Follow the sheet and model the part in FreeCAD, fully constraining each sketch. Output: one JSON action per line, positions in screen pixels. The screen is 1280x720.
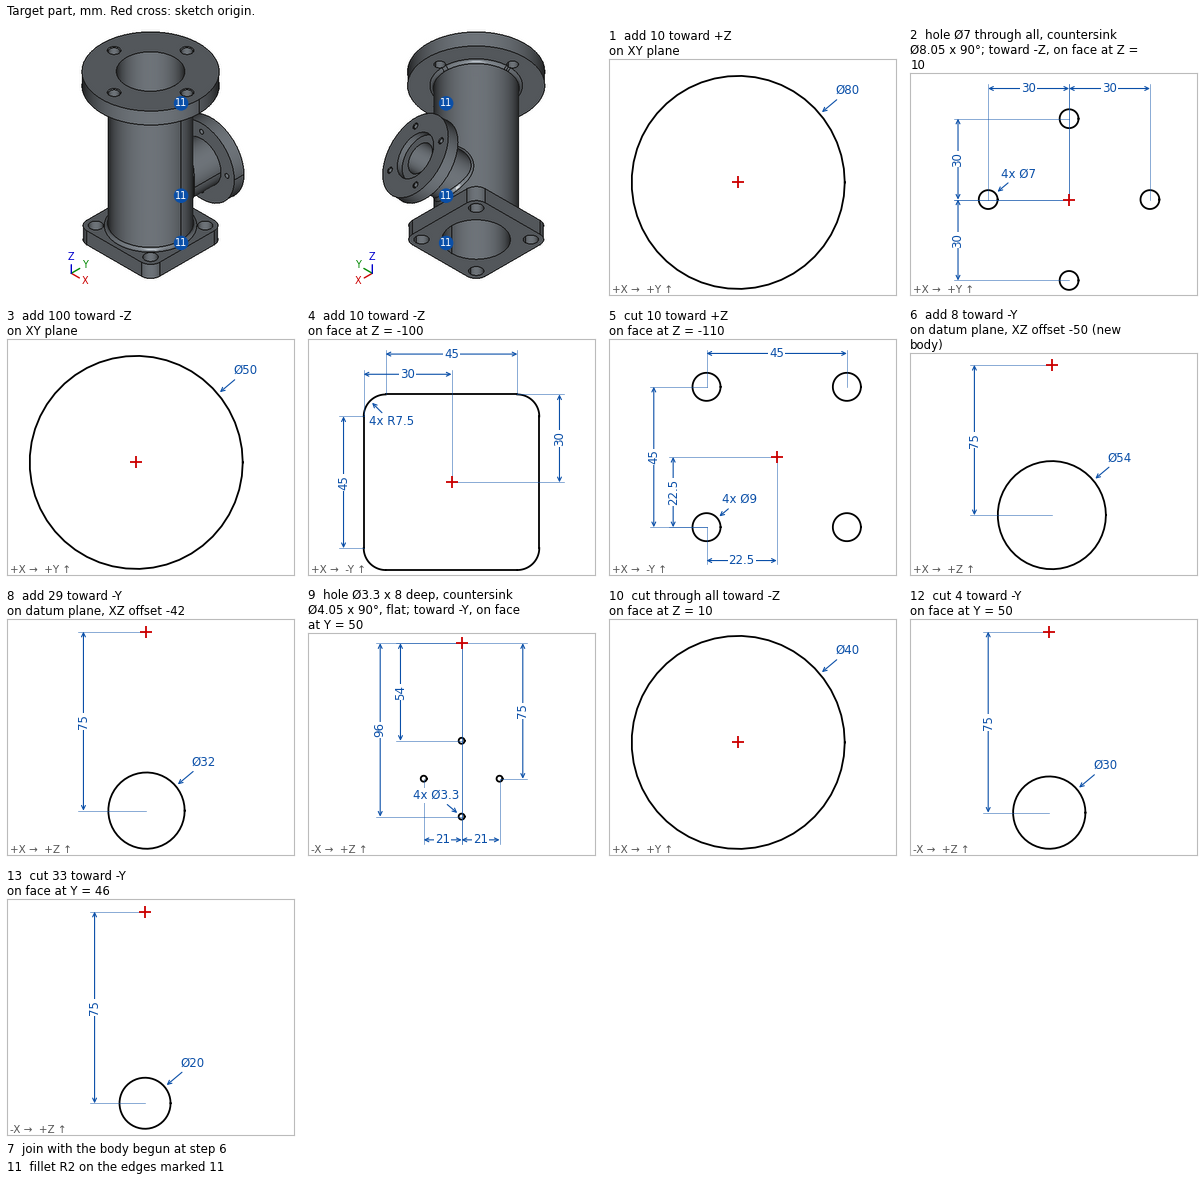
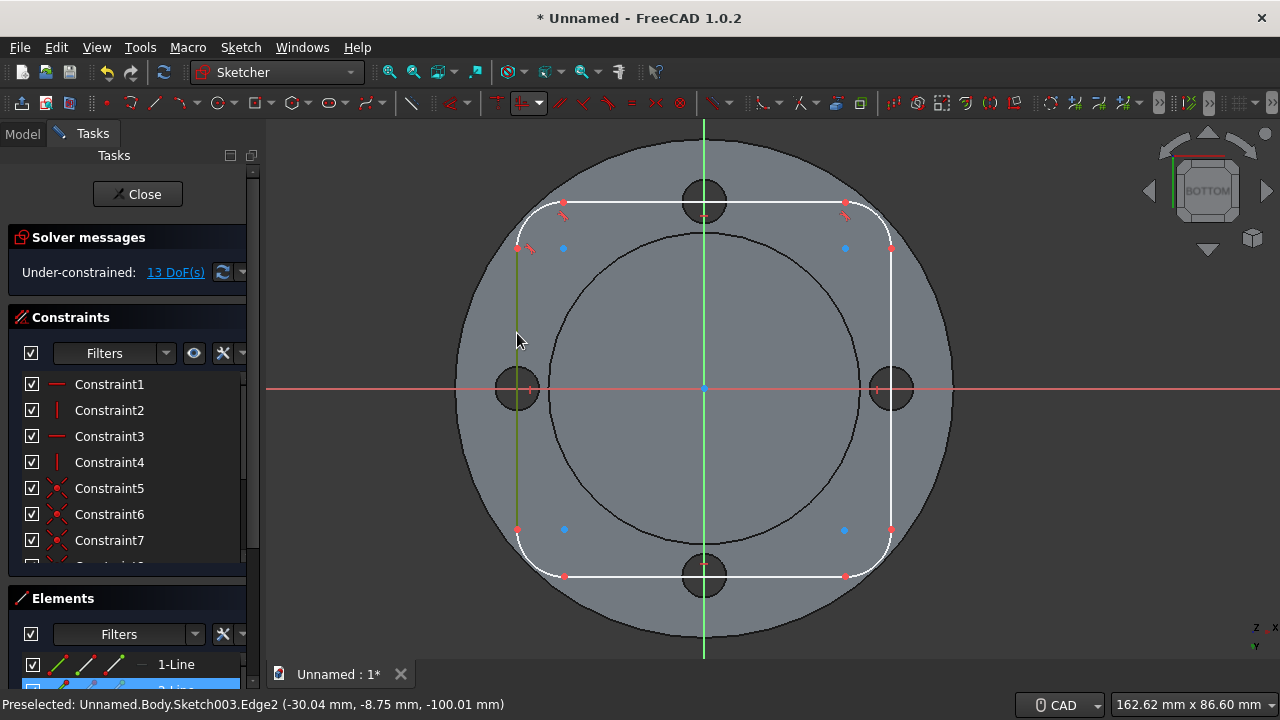
{"action": "left_click", "coordinate": [522, 551]}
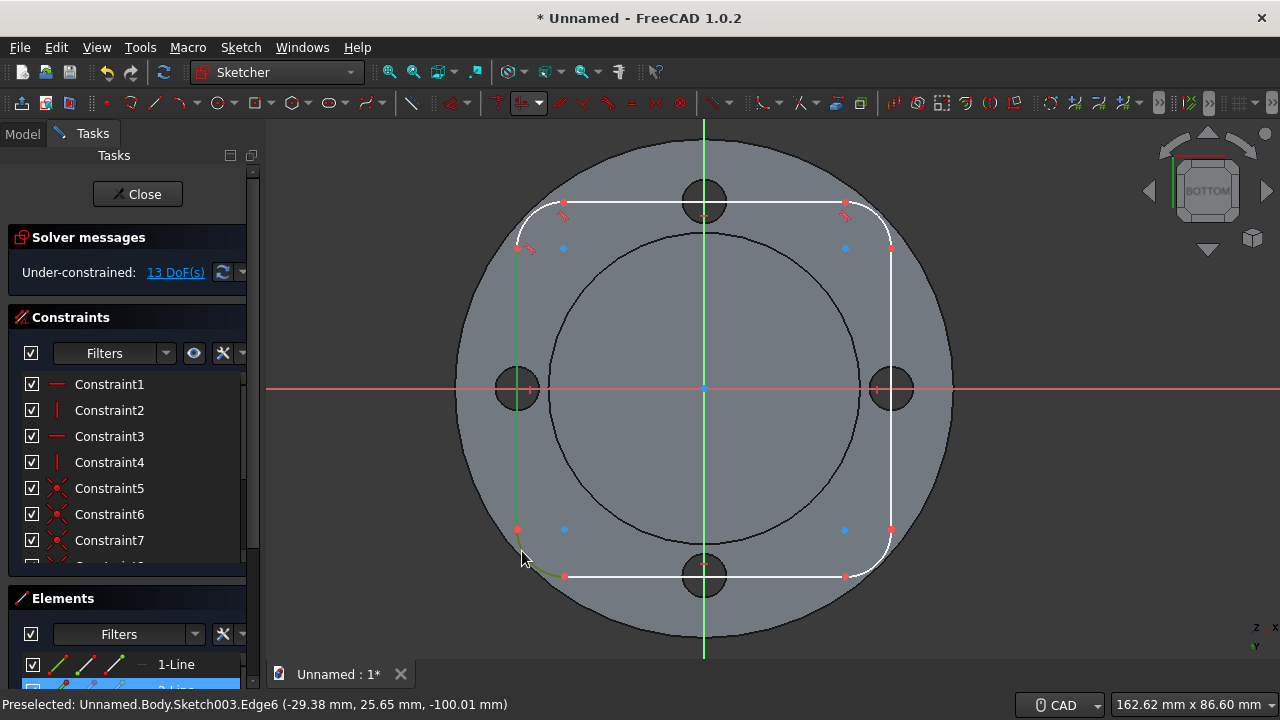
{"action": "left_click", "coordinate": [608, 104]}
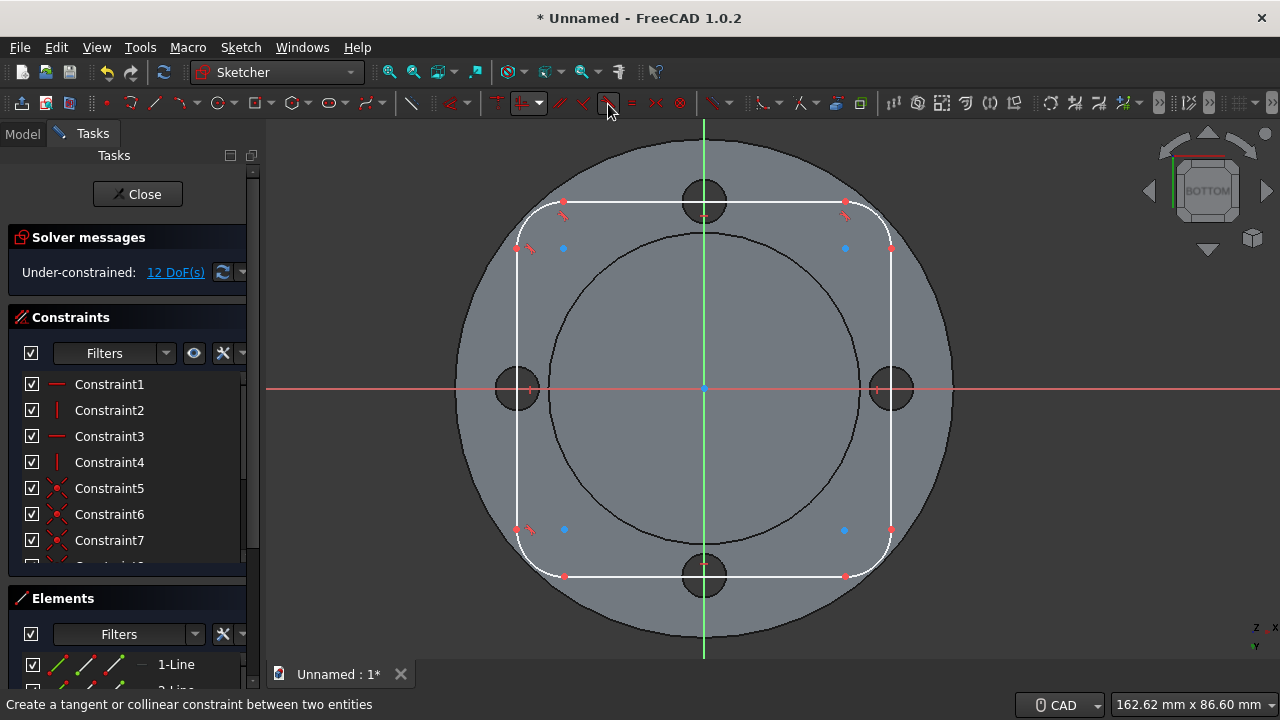
{"action": "left_click", "coordinate": [648, 577]}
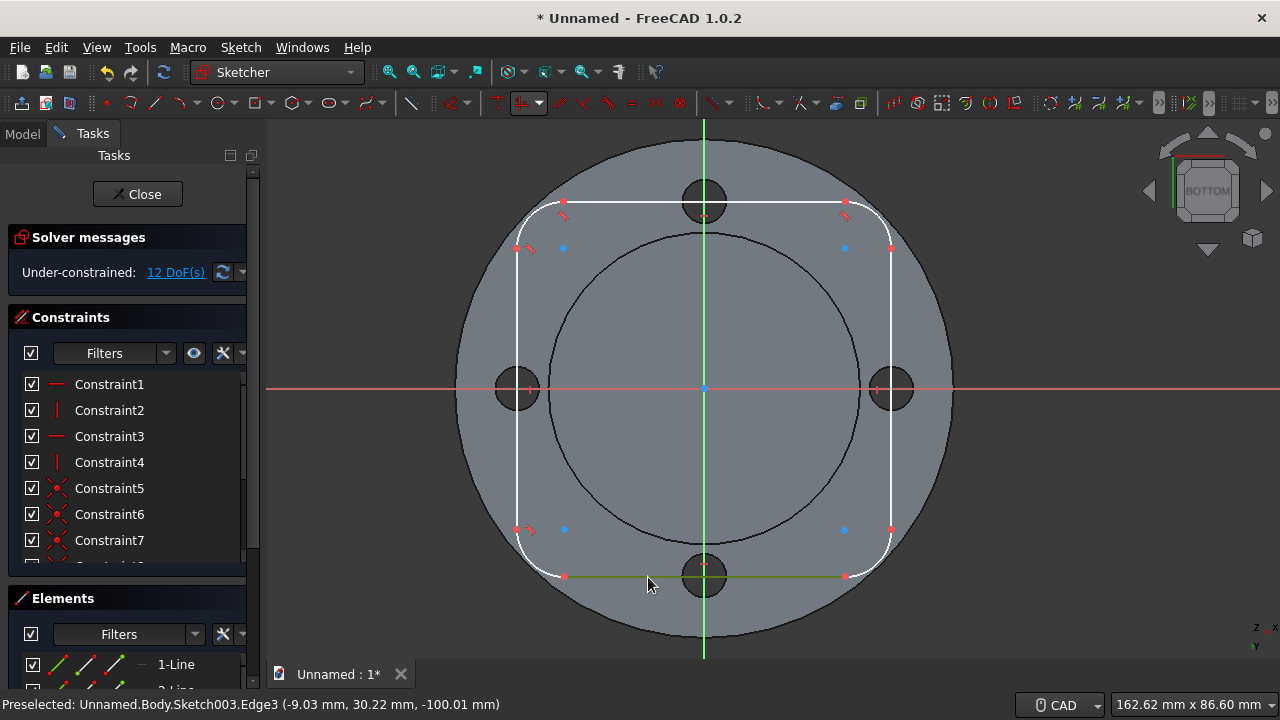
{"action": "left_click", "coordinate": [522, 551]}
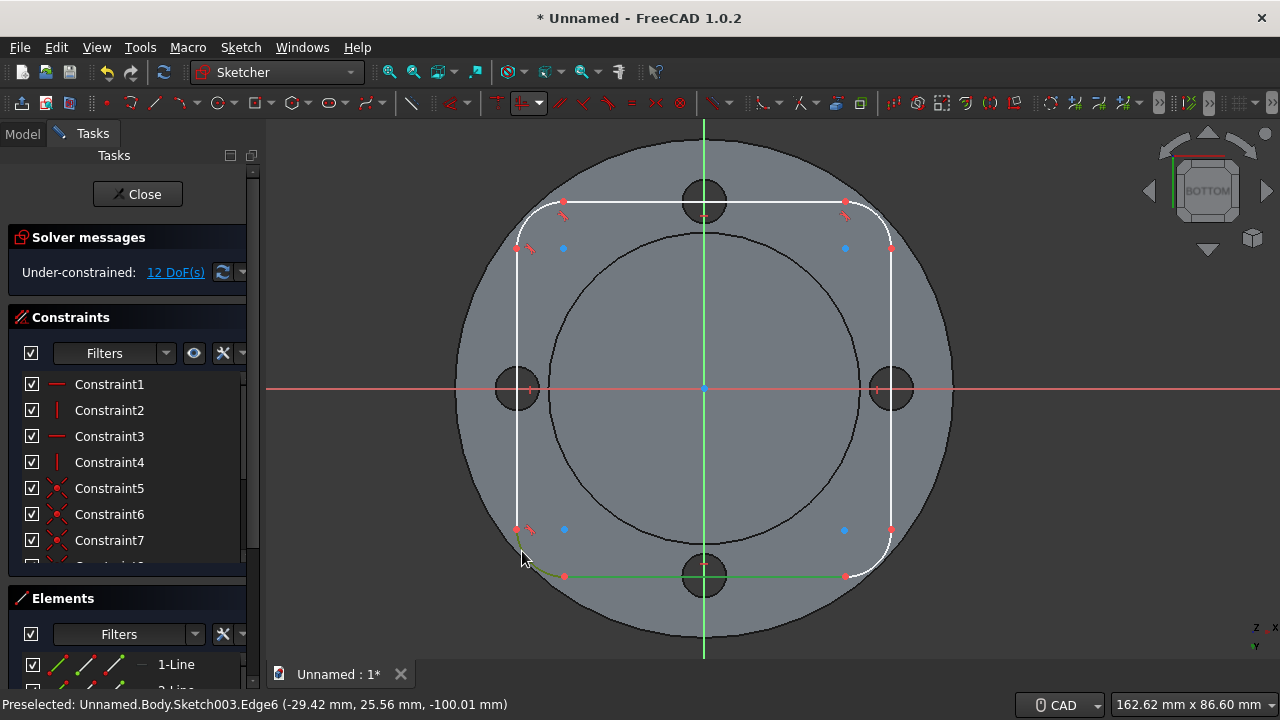
{"action": "left_click", "coordinate": [608, 104]}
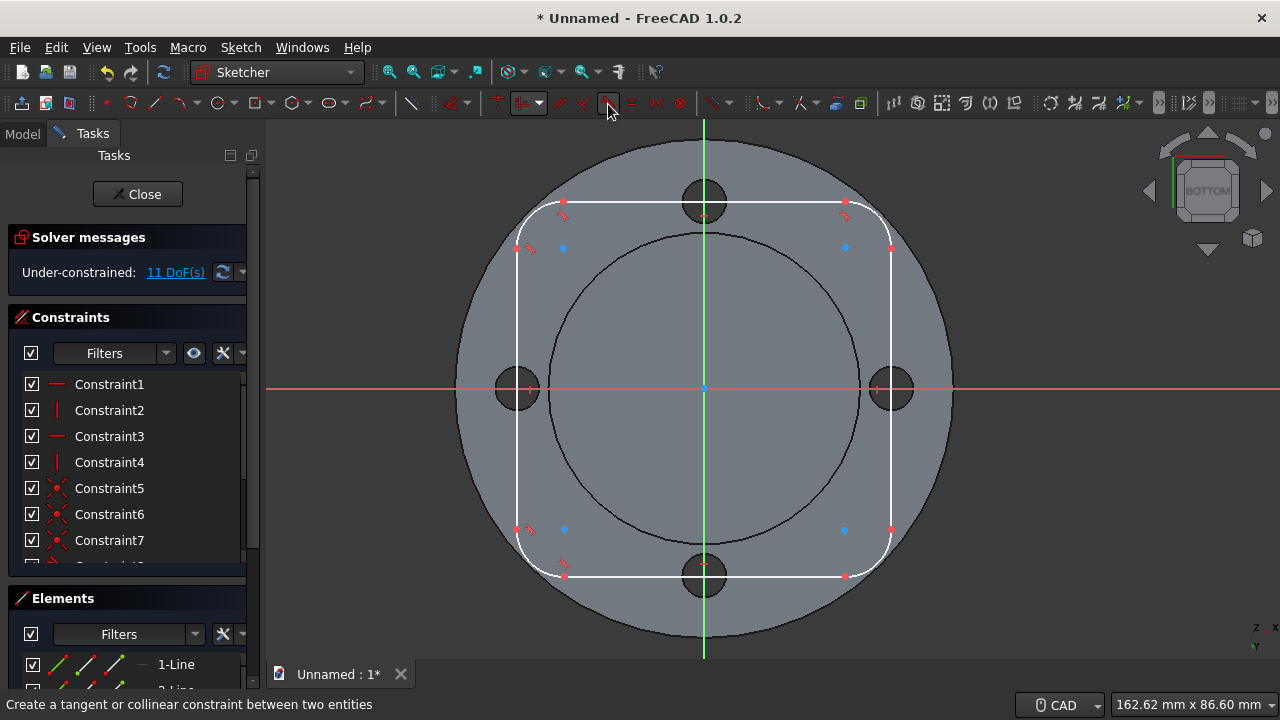
{"action": "left_click", "coordinate": [649, 577]}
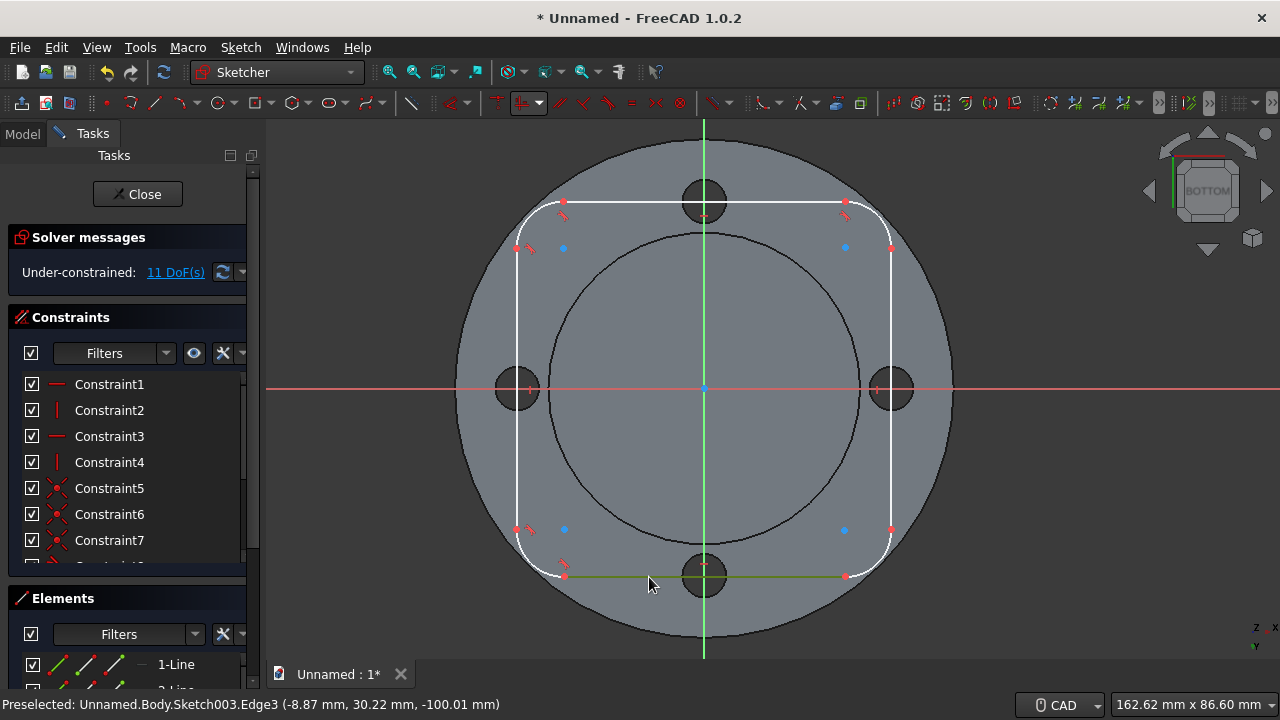
{"action": "left_click", "coordinate": [866, 572]}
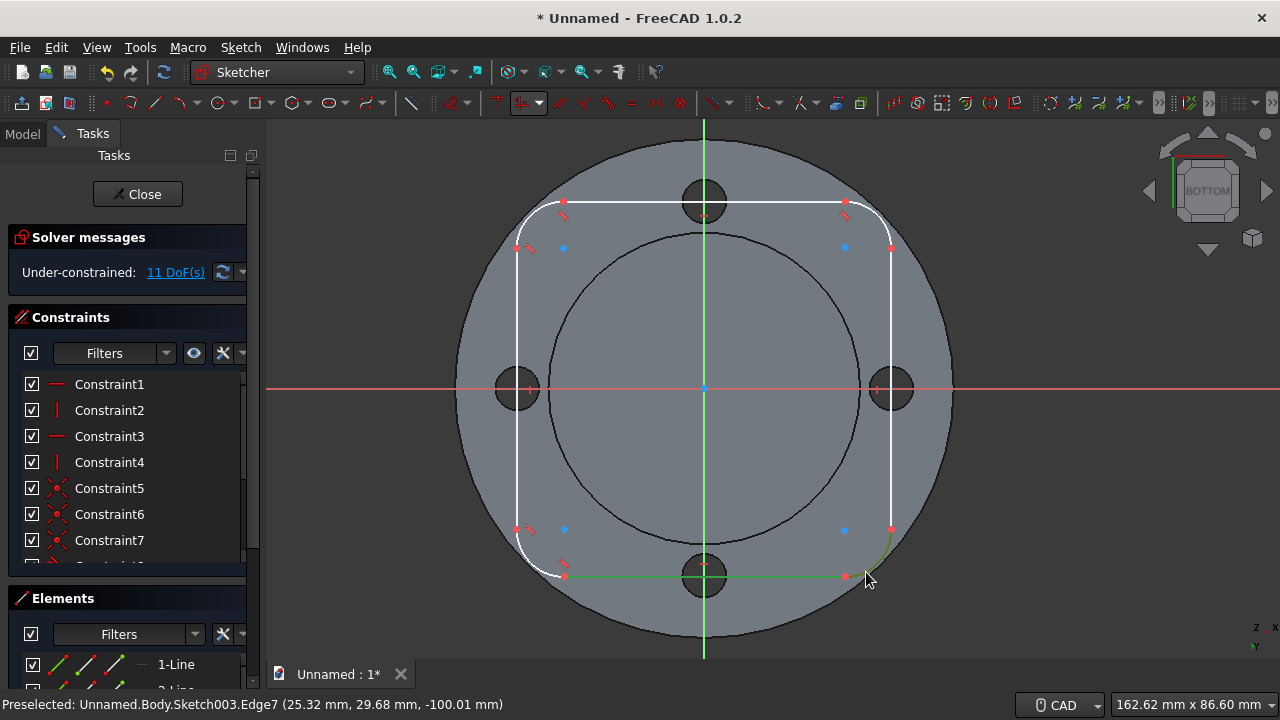
{"action": "left_click", "coordinate": [608, 104]}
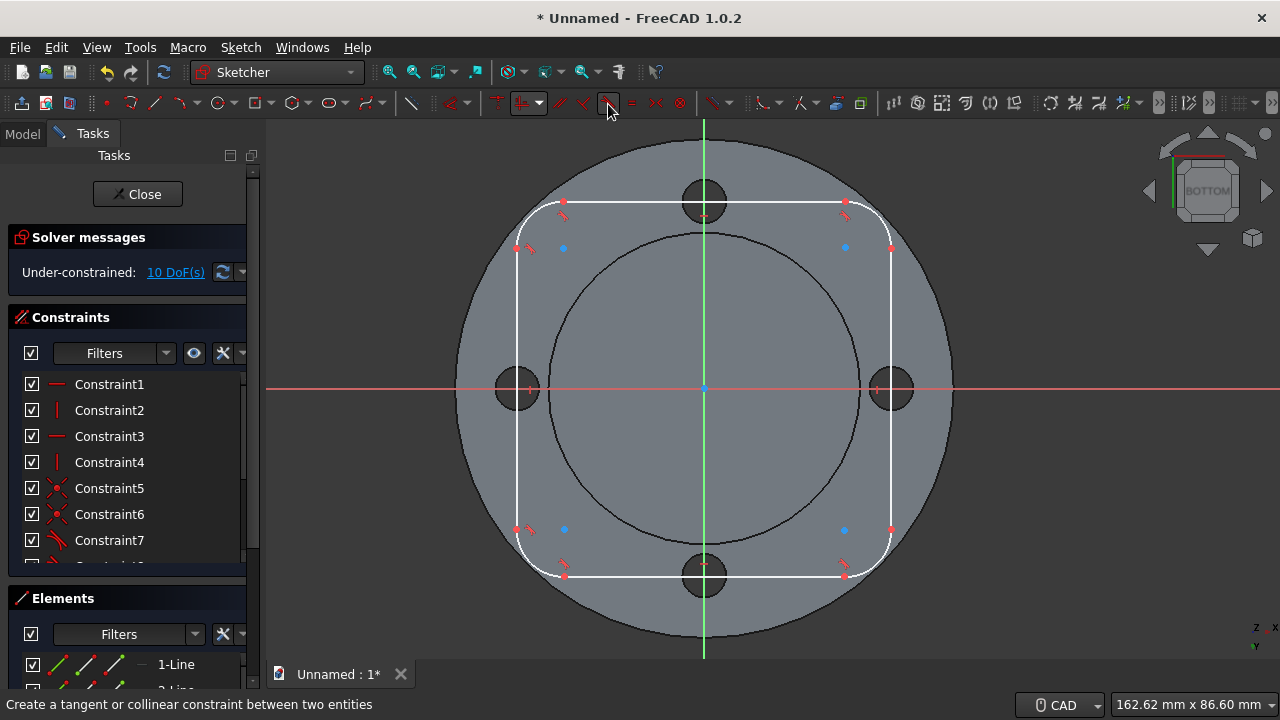
{"action": "left_click", "coordinate": [891, 446]}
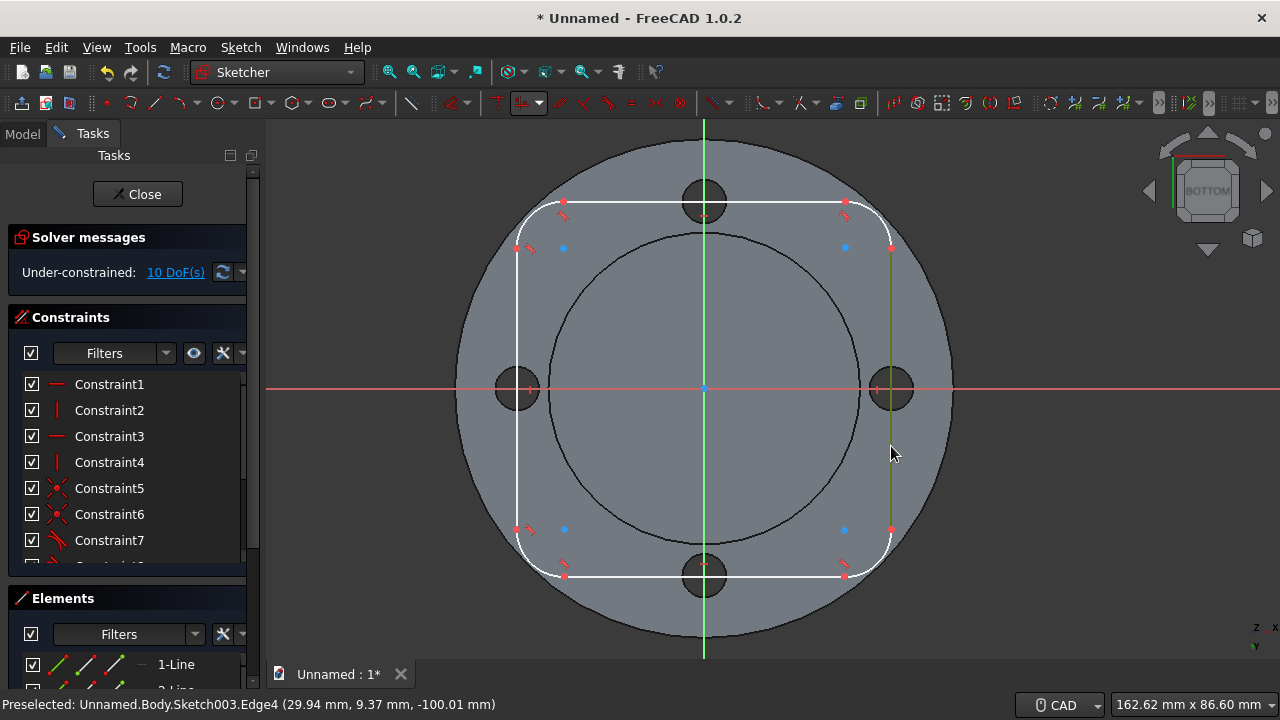
{"action": "left_click", "coordinate": [866, 572]}